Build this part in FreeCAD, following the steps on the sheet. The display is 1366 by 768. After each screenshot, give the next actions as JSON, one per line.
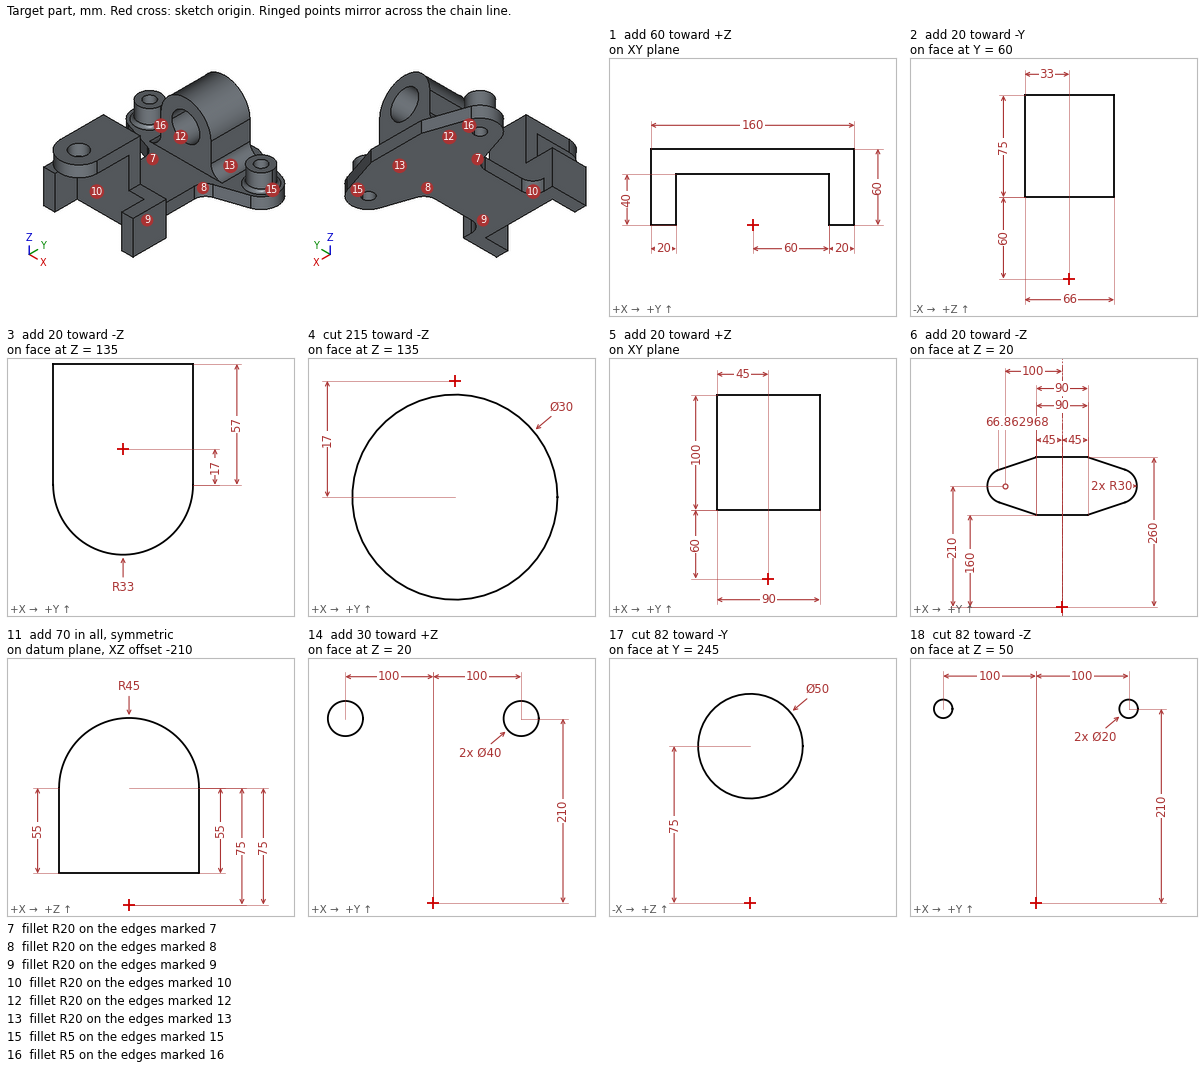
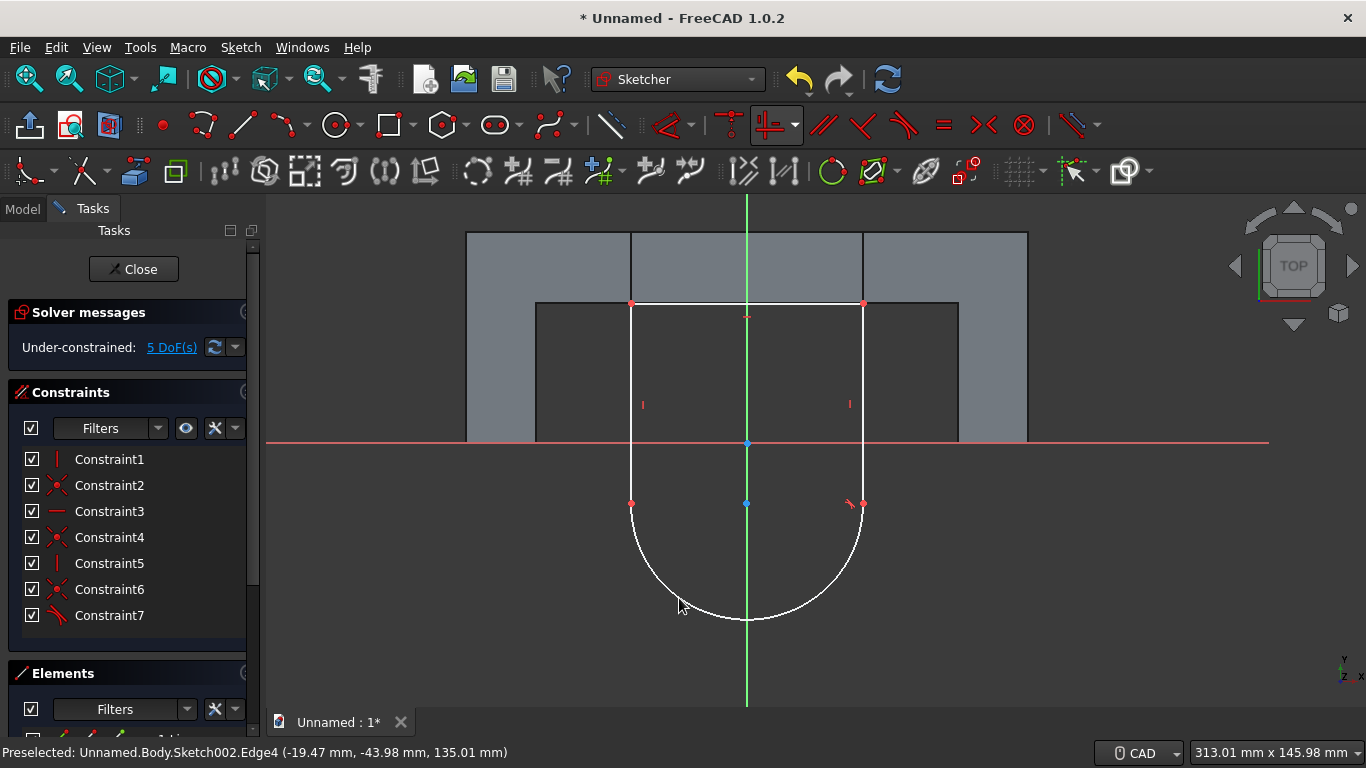
{"action": "left_click", "coordinate": [631, 364]}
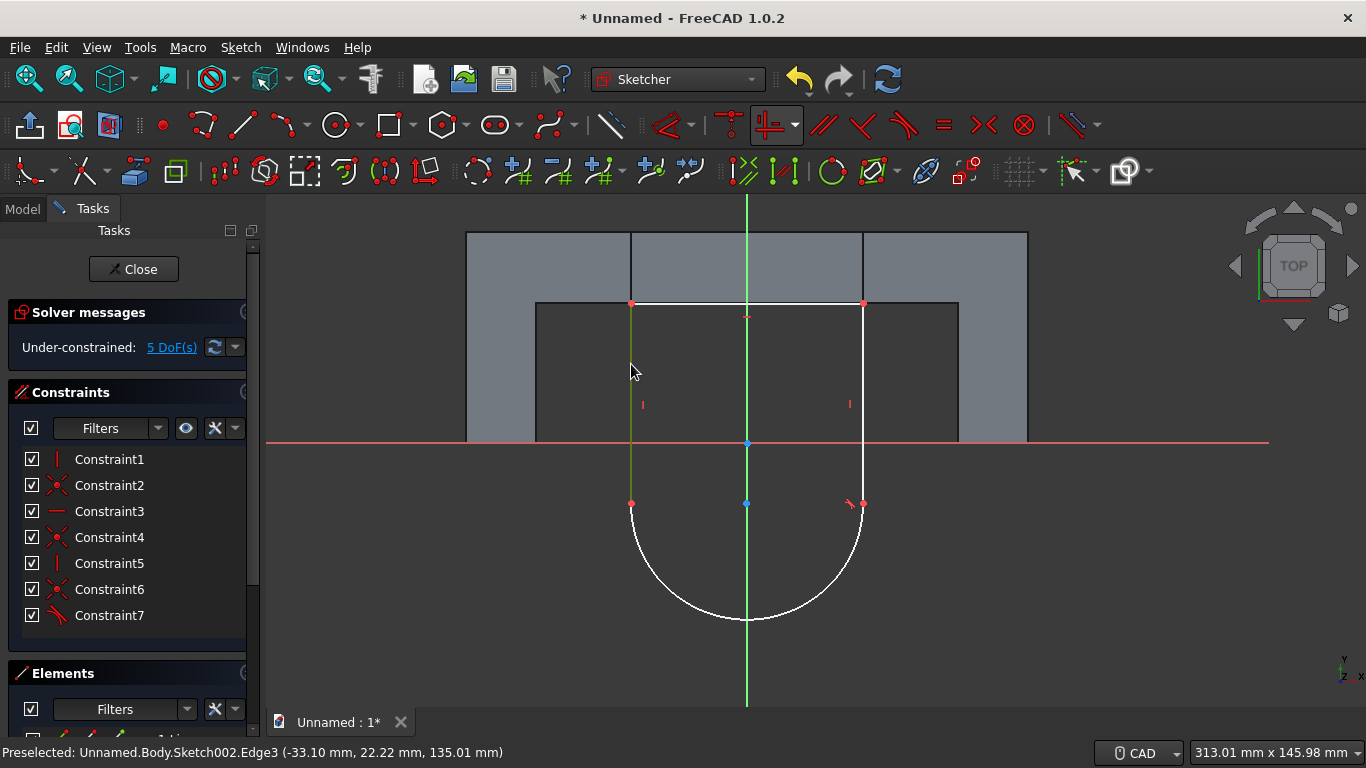
{"action": "left_click", "coordinate": [679, 598]}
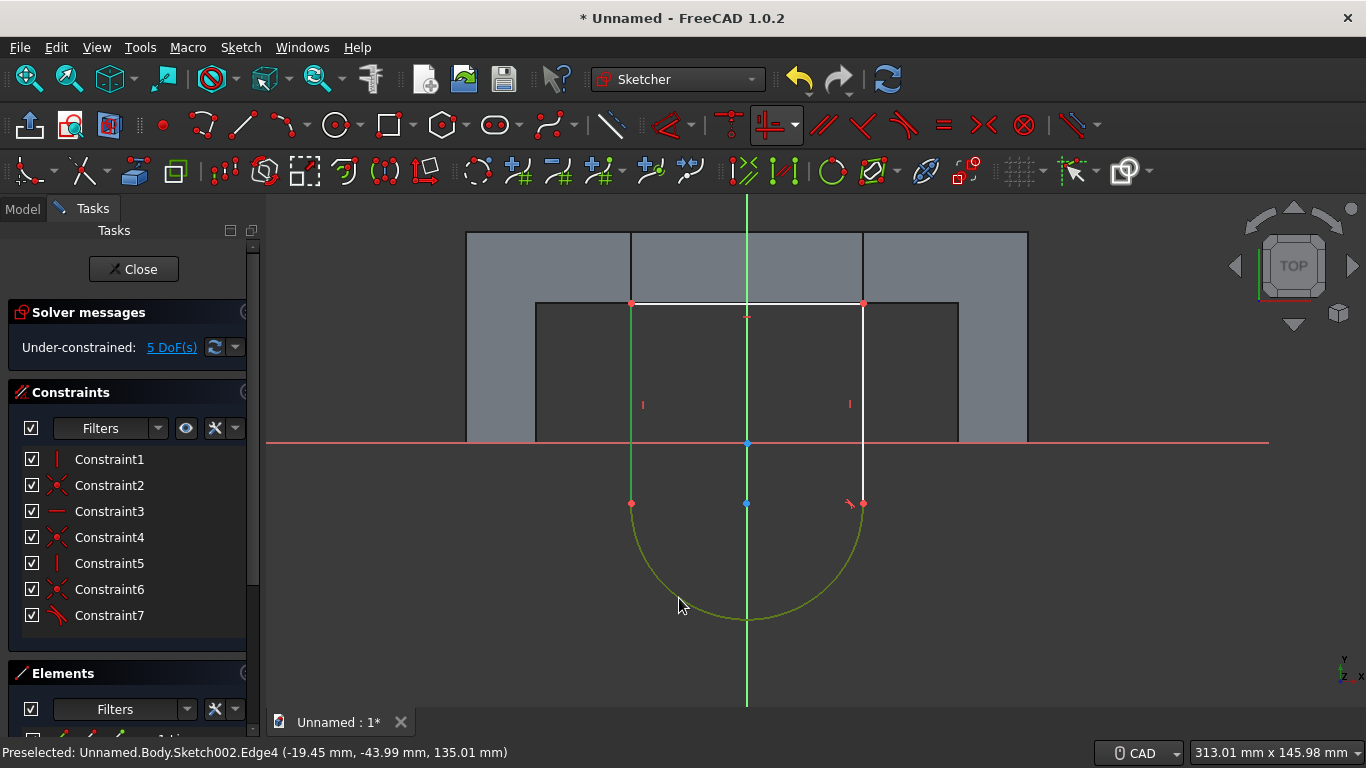
{"action": "key", "text": "t"}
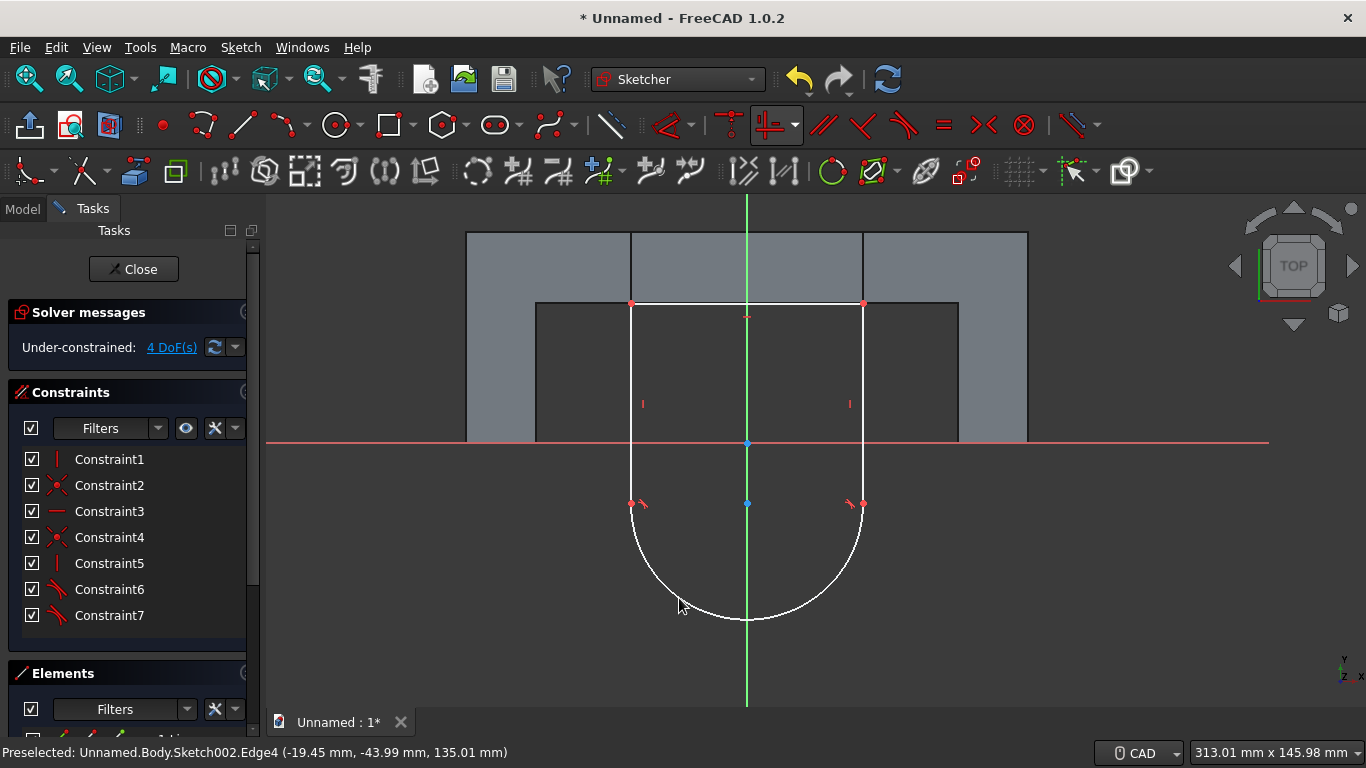
{"action": "left_click", "coordinate": [747, 504]}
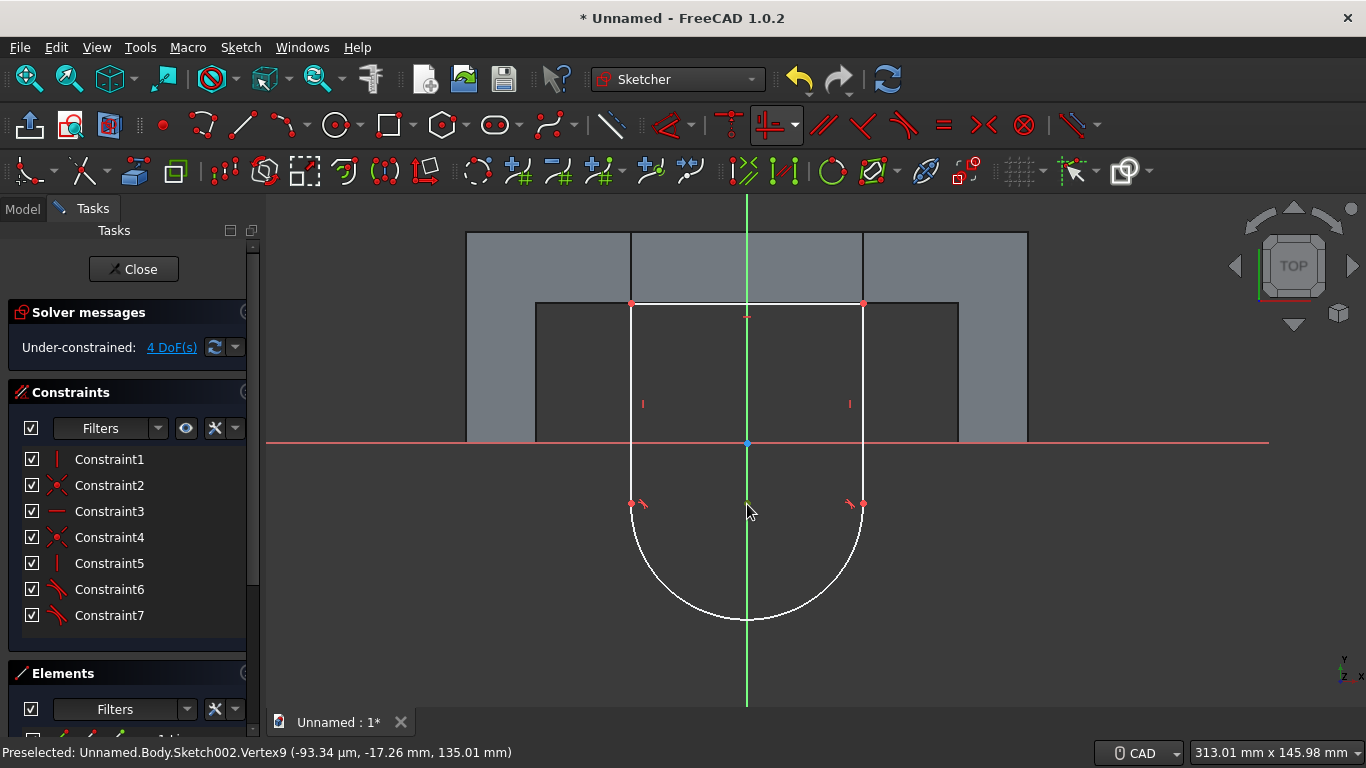
{"action": "left_click", "coordinate": [747, 581]}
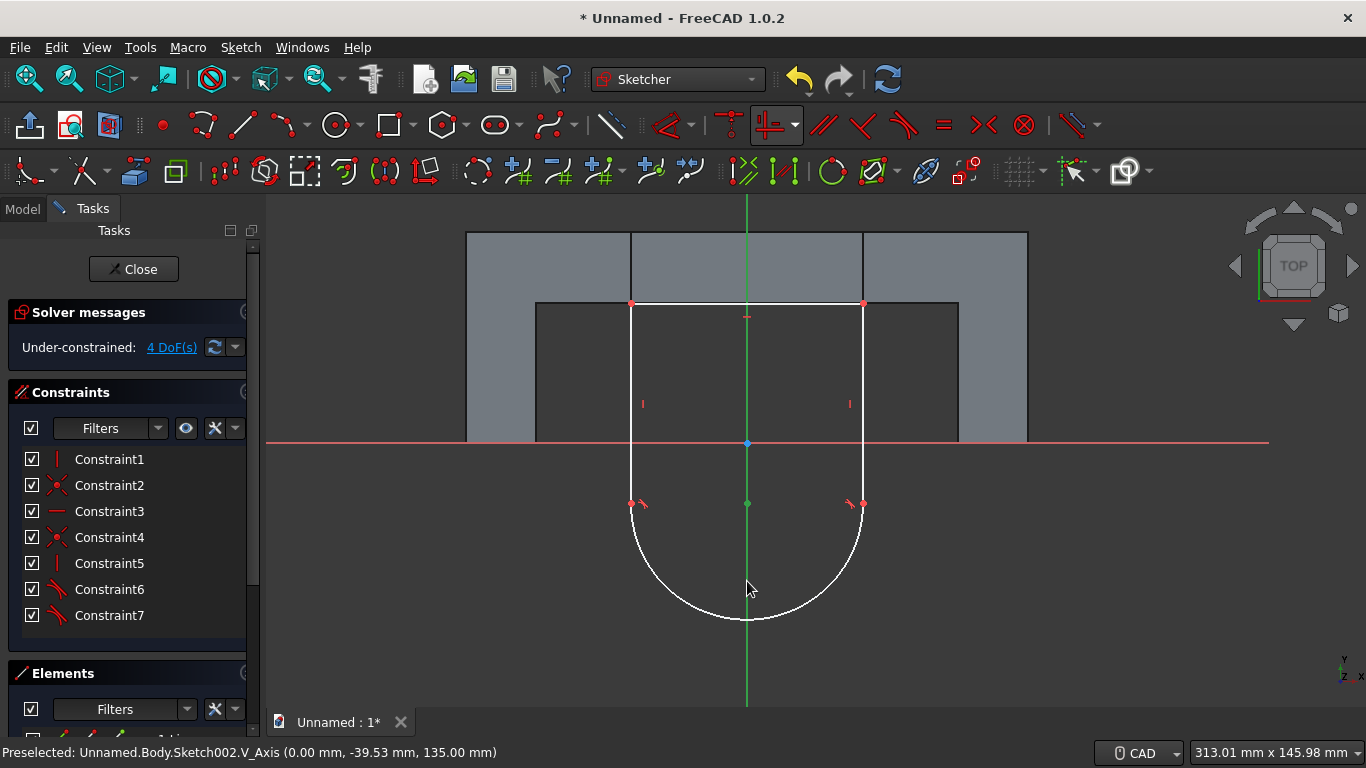
{"action": "key", "text": "c"}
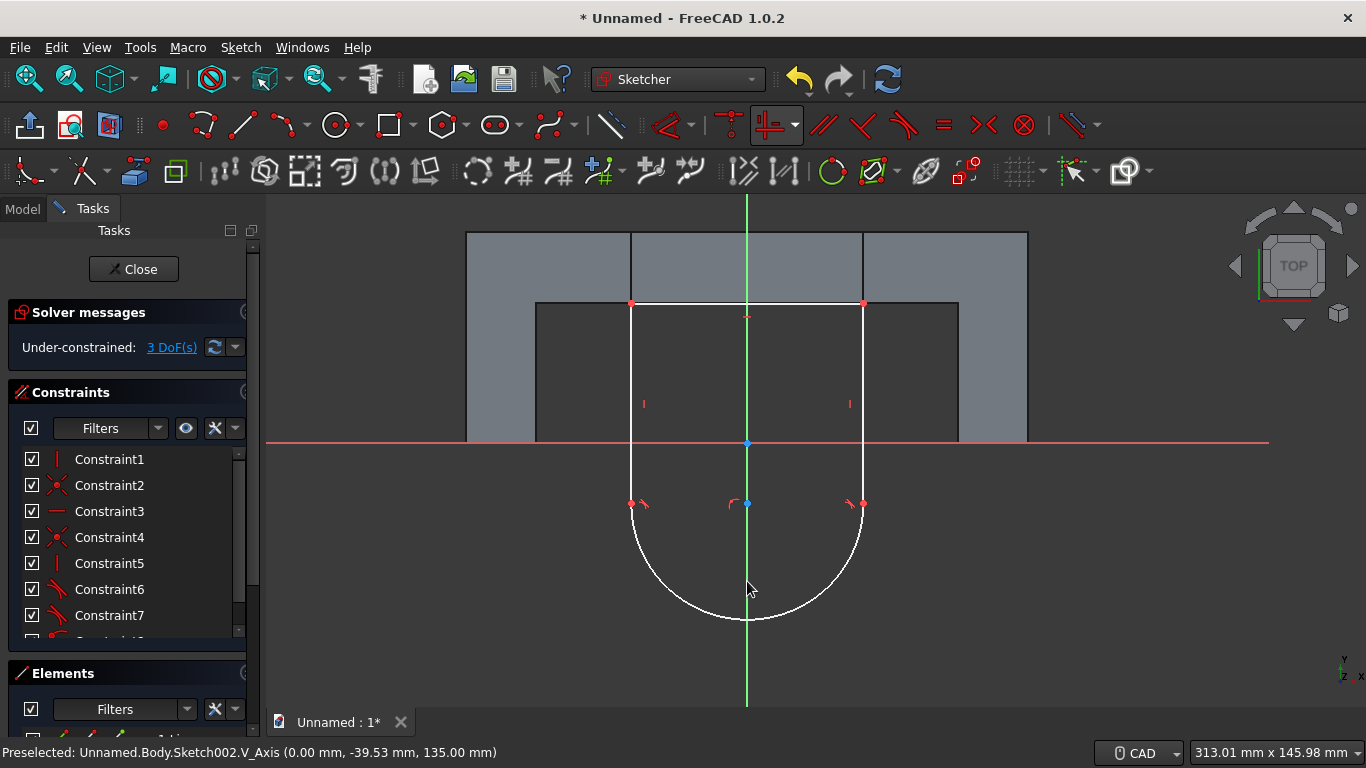
{"action": "key", "text": "d"}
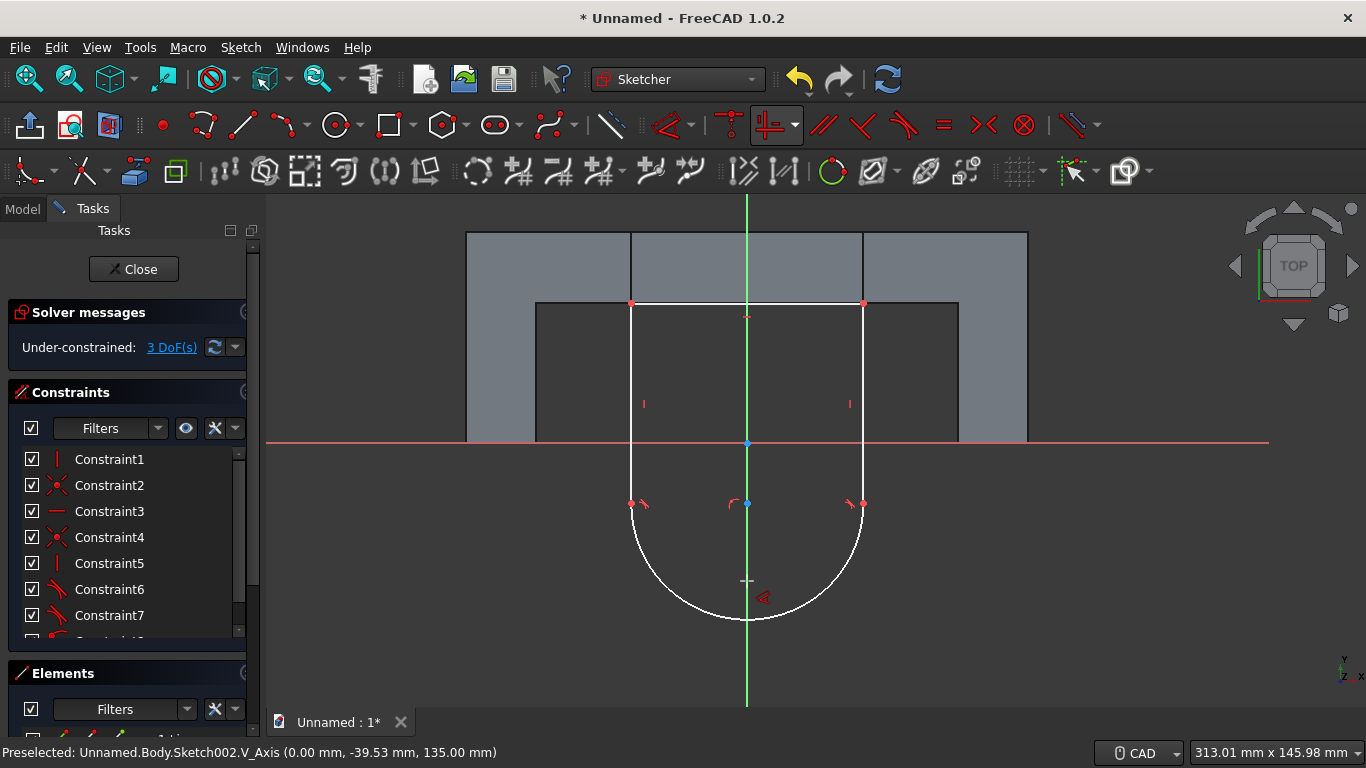
{"action": "left_click", "coordinate": [679, 598]}
{"action": "left_click", "coordinate": [660, 624]}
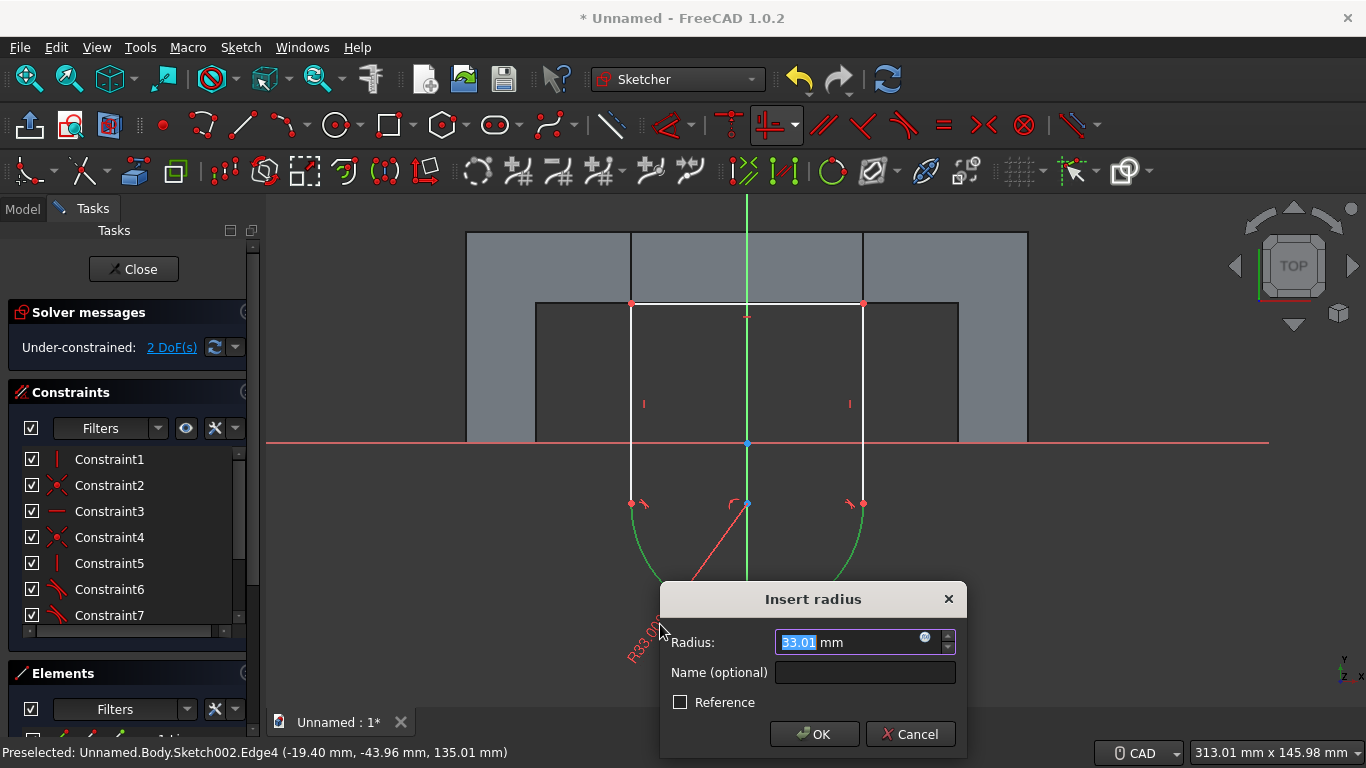
{"action": "type", "text": "33"}
{"action": "key", "text": "Return"}